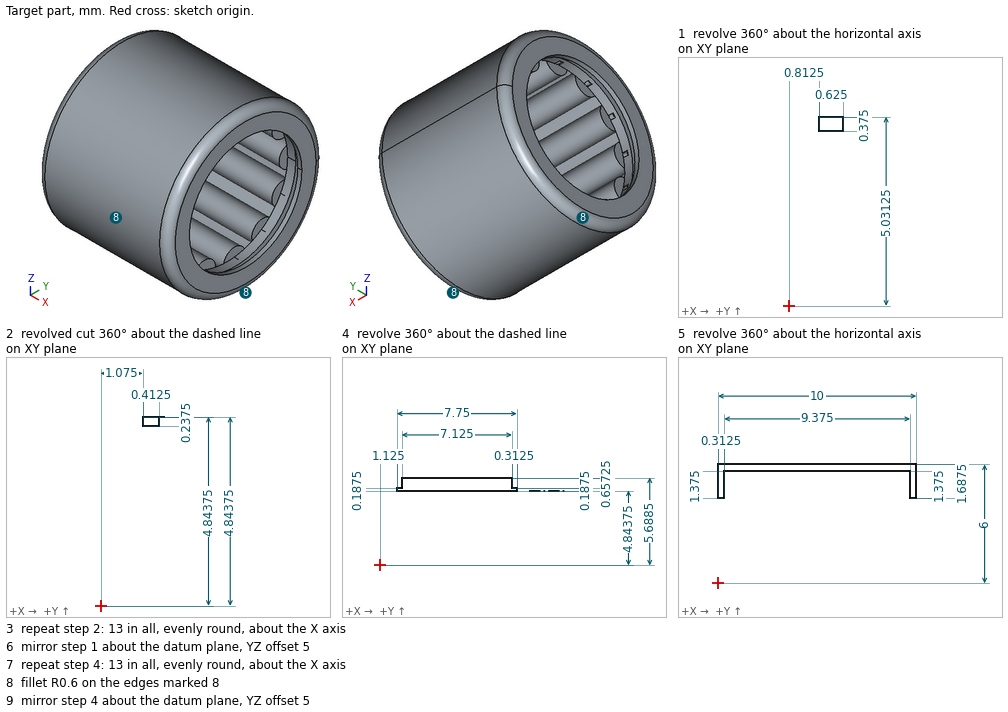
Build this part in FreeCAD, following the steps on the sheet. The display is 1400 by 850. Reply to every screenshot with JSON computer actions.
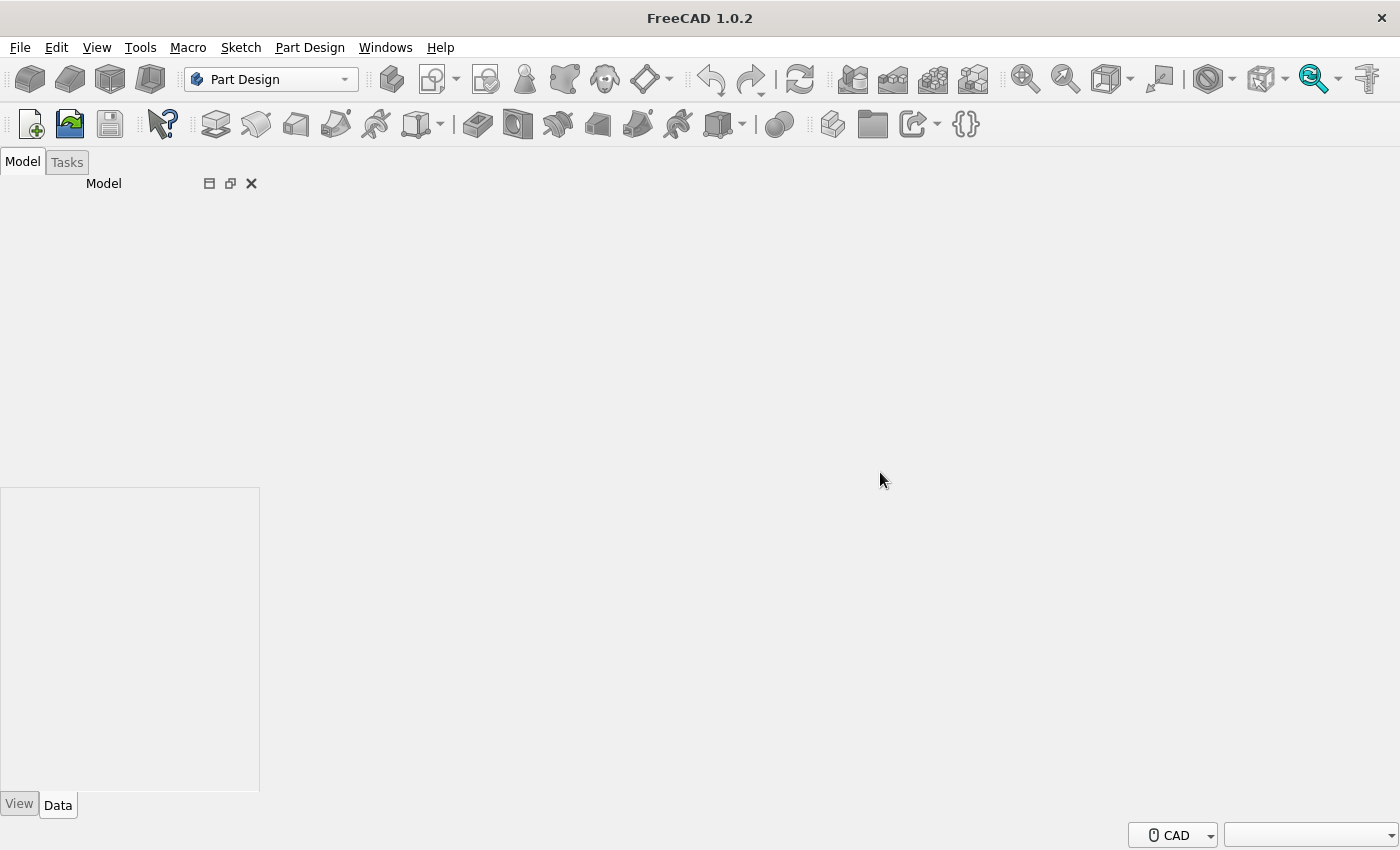
{"action": "key", "text": "ctrl+n"}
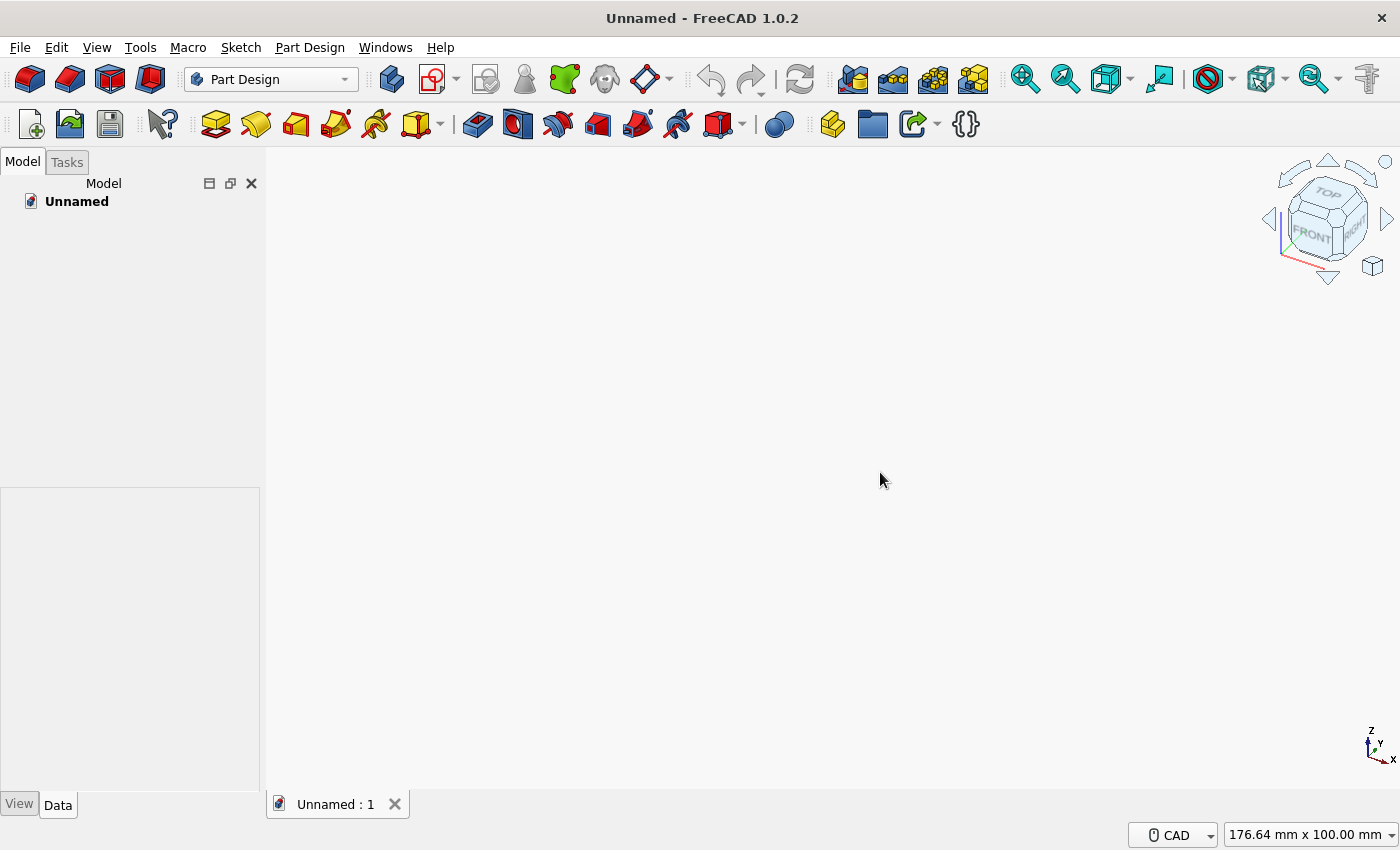
{"action": "left_click", "coordinate": [432, 80]}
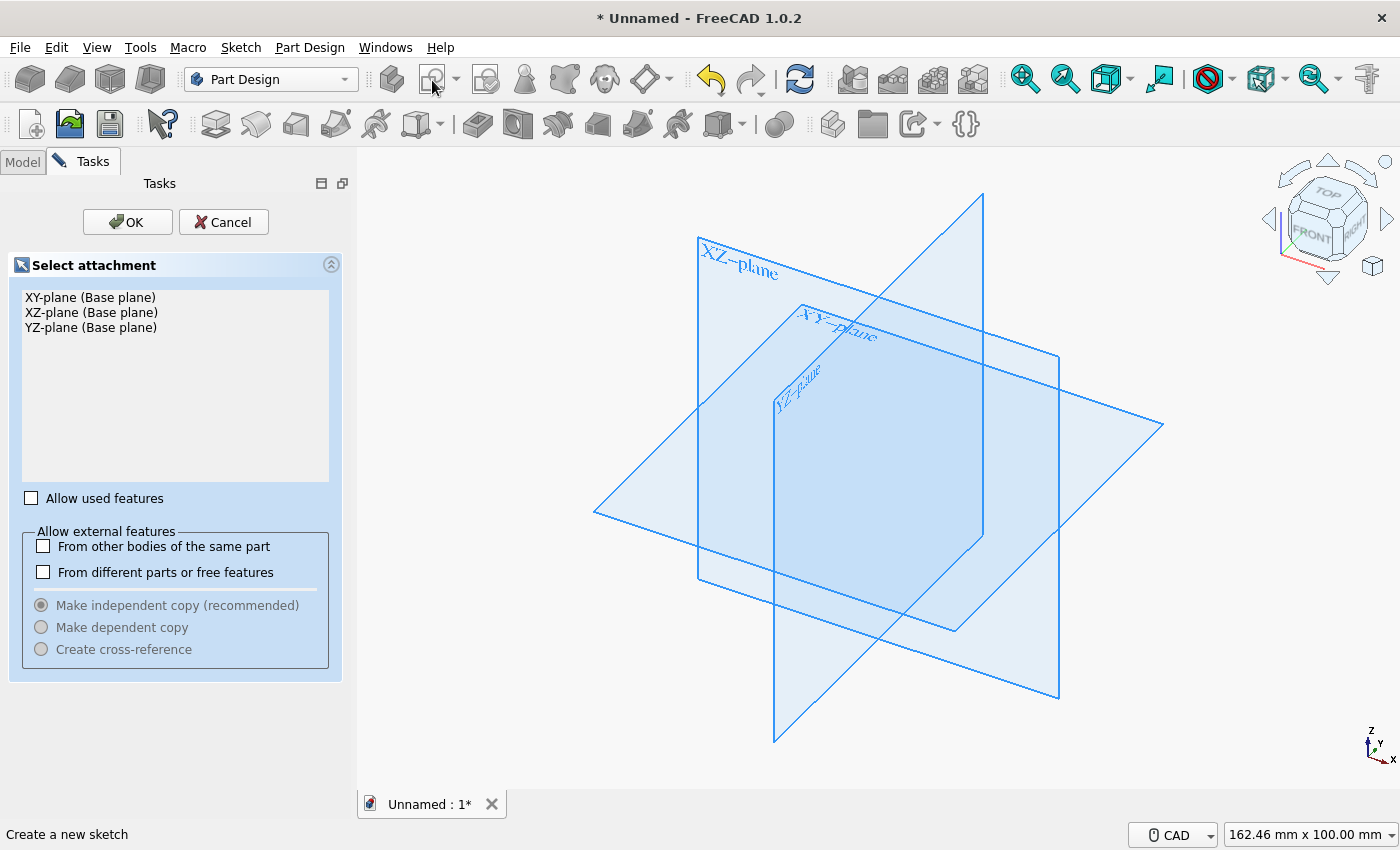
{"action": "left_click", "coordinate": [82, 298]}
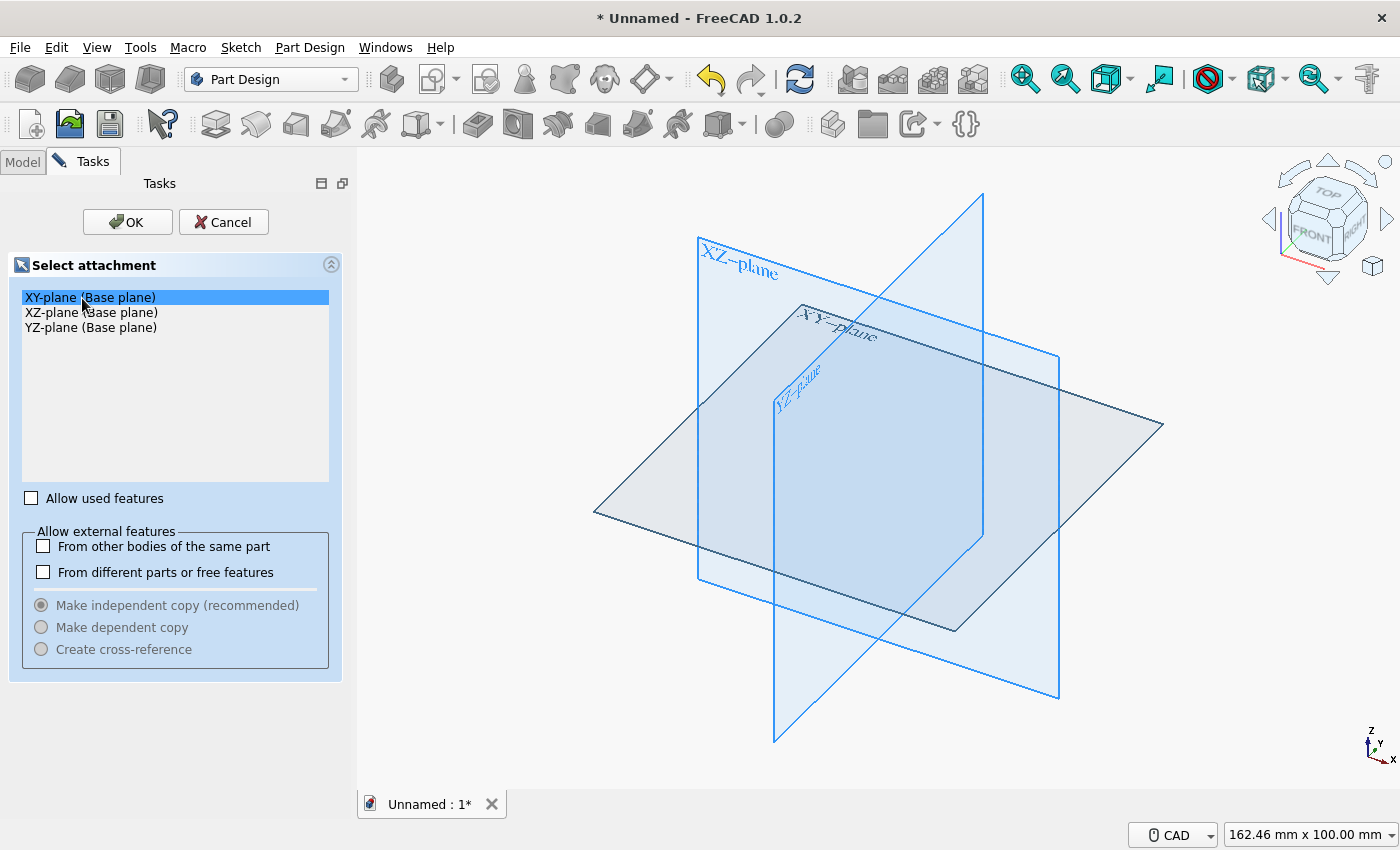
{"action": "left_click", "coordinate": [128, 222]}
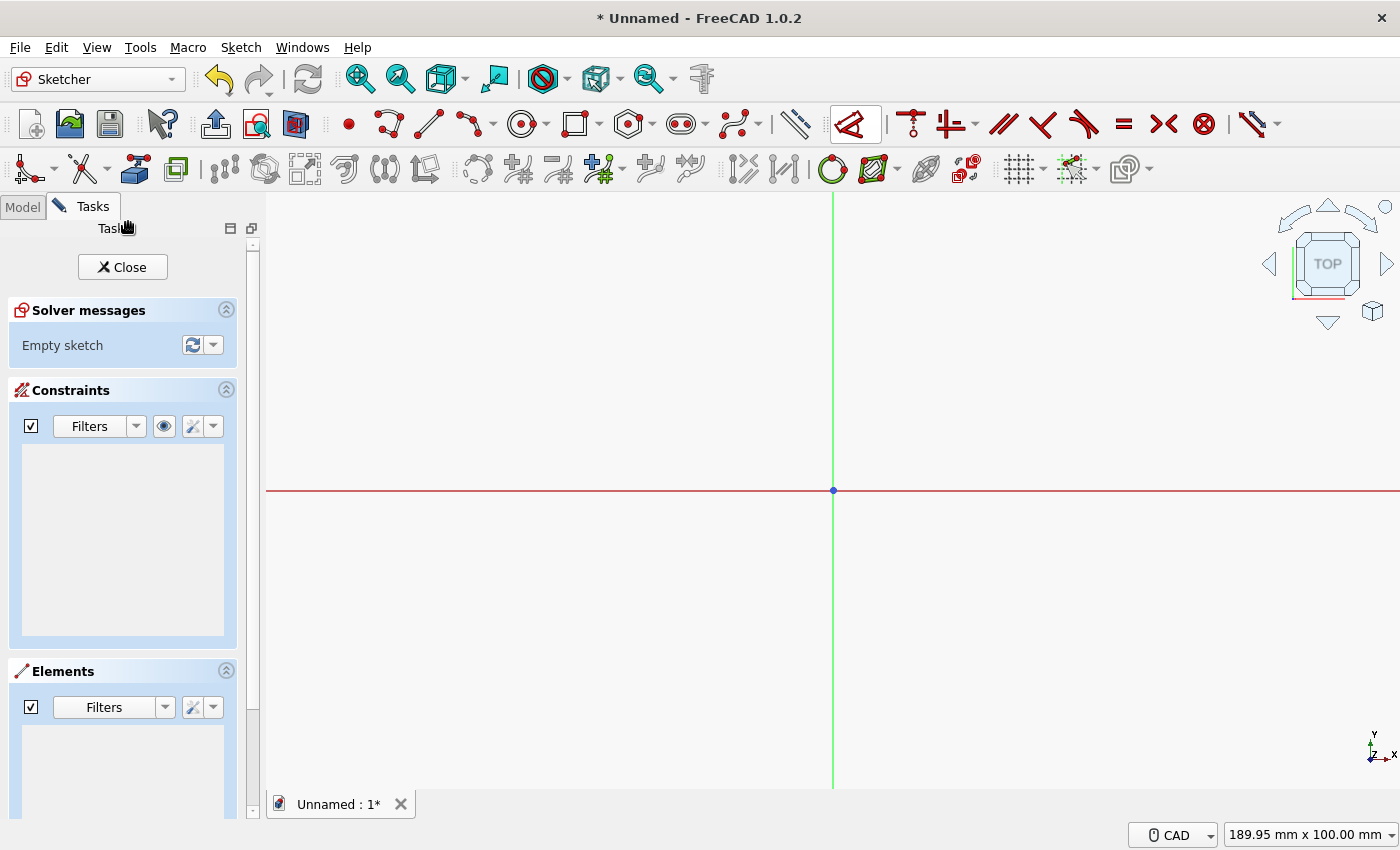
{"action": "scroll", "coordinate": [844, 460], "scroll_direction": "up", "scroll_amount": 15}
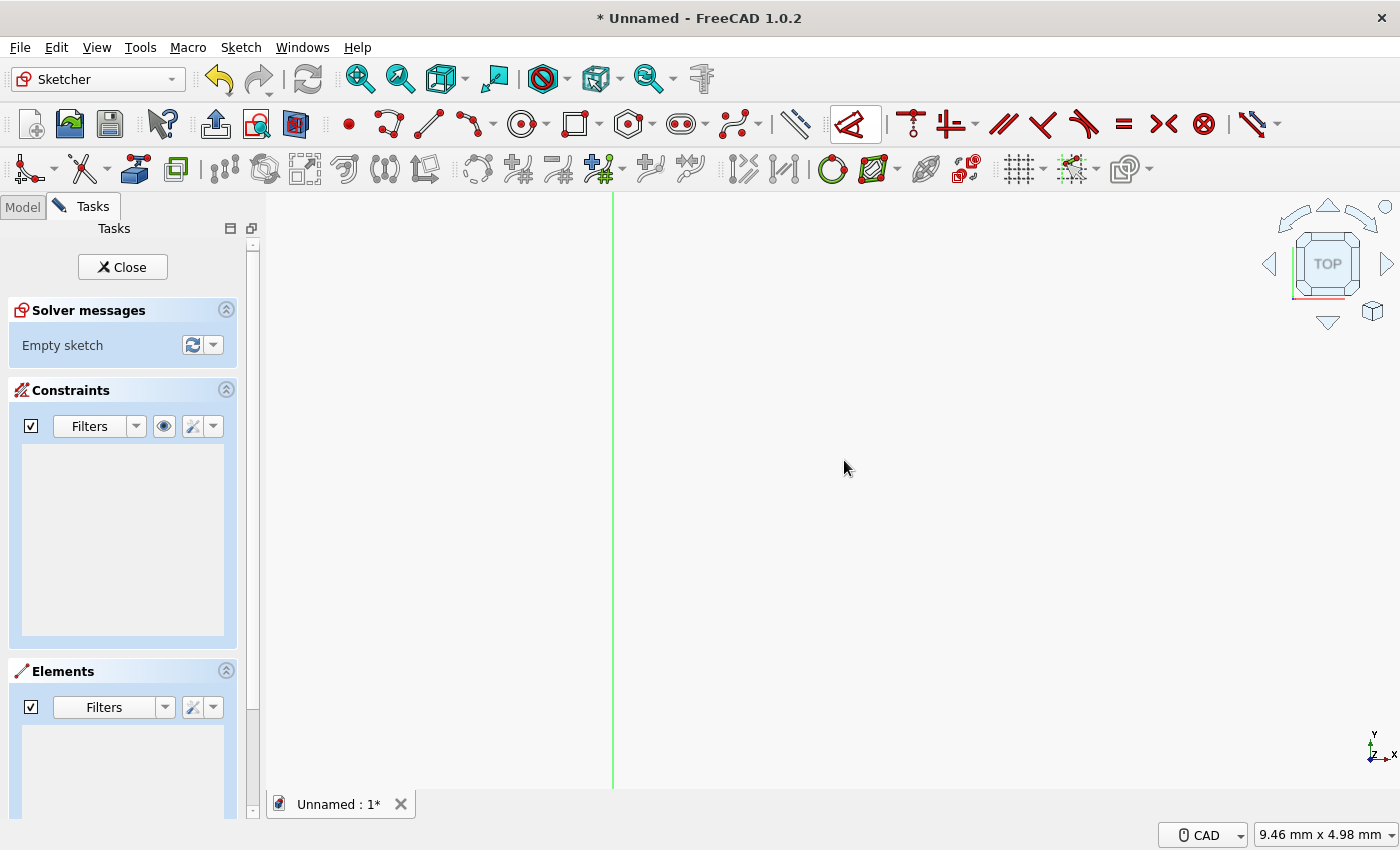
{"action": "scroll", "coordinate": [746, 482], "scroll_direction": "up", "scroll_amount": 11}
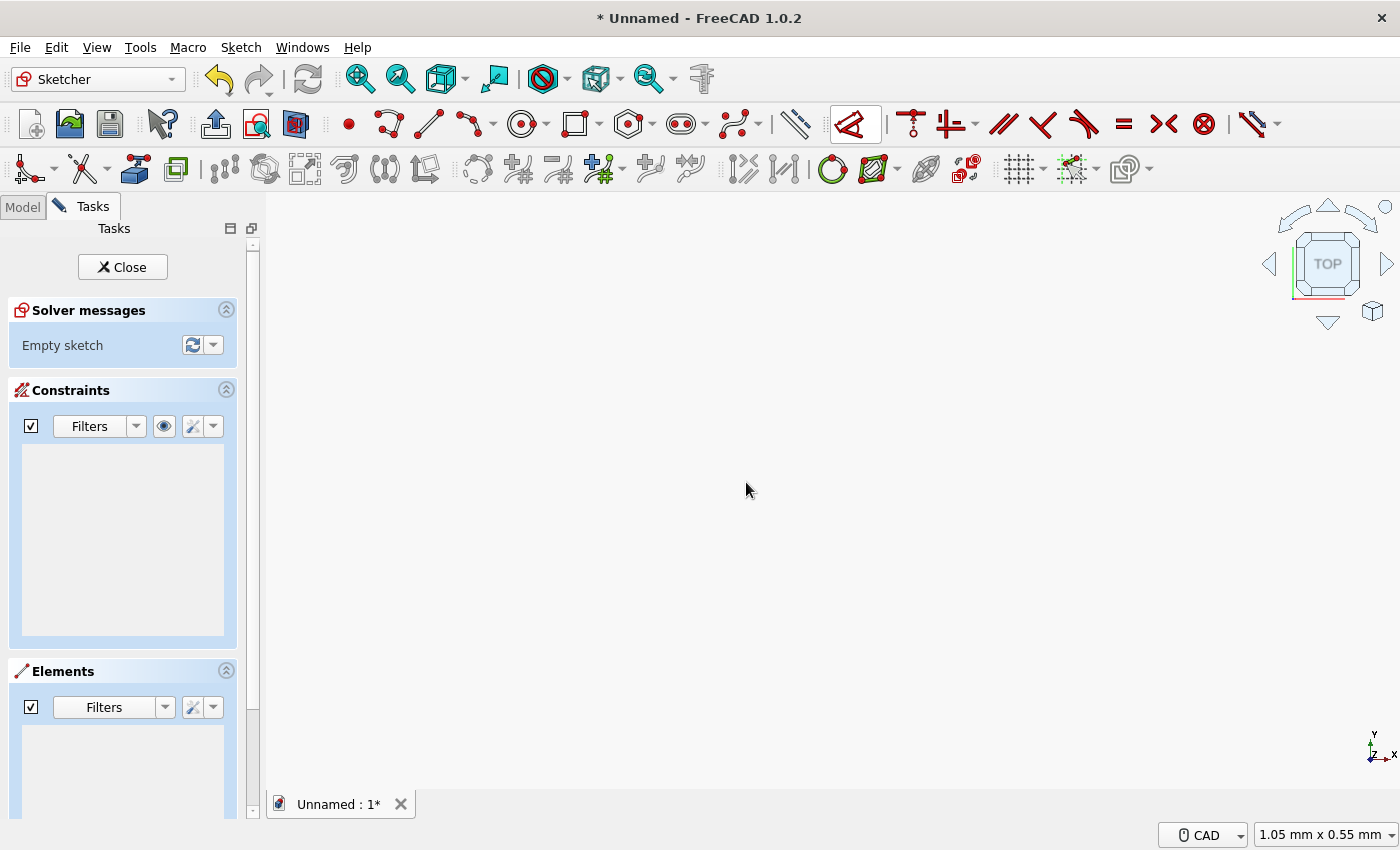
{"action": "left_click", "coordinate": [576, 124]}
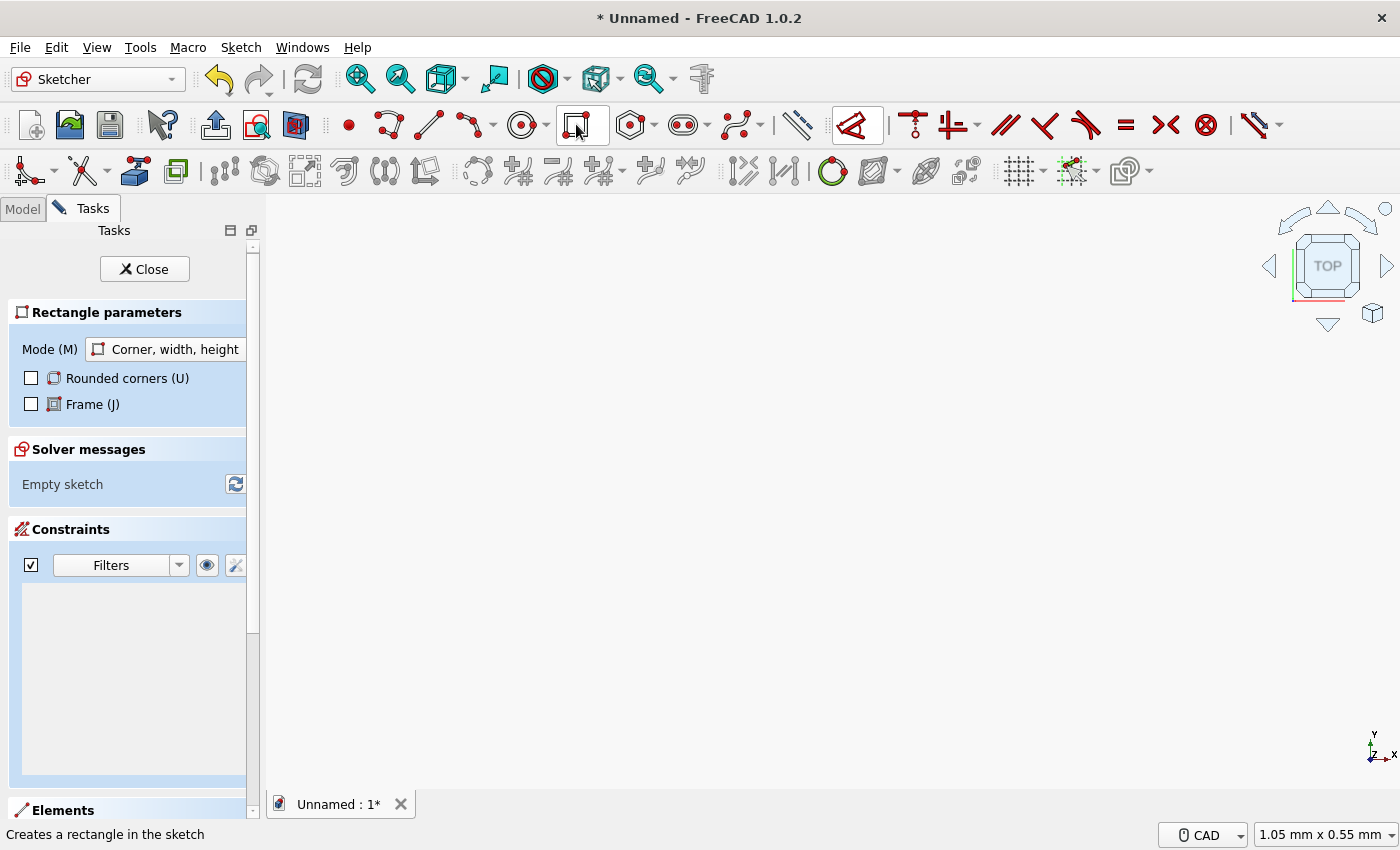
{"action": "left_click", "coordinate": [426, 288]}
{"action": "left_click", "coordinate": [1100, 692]}
{"action": "key", "text": "Escape"}